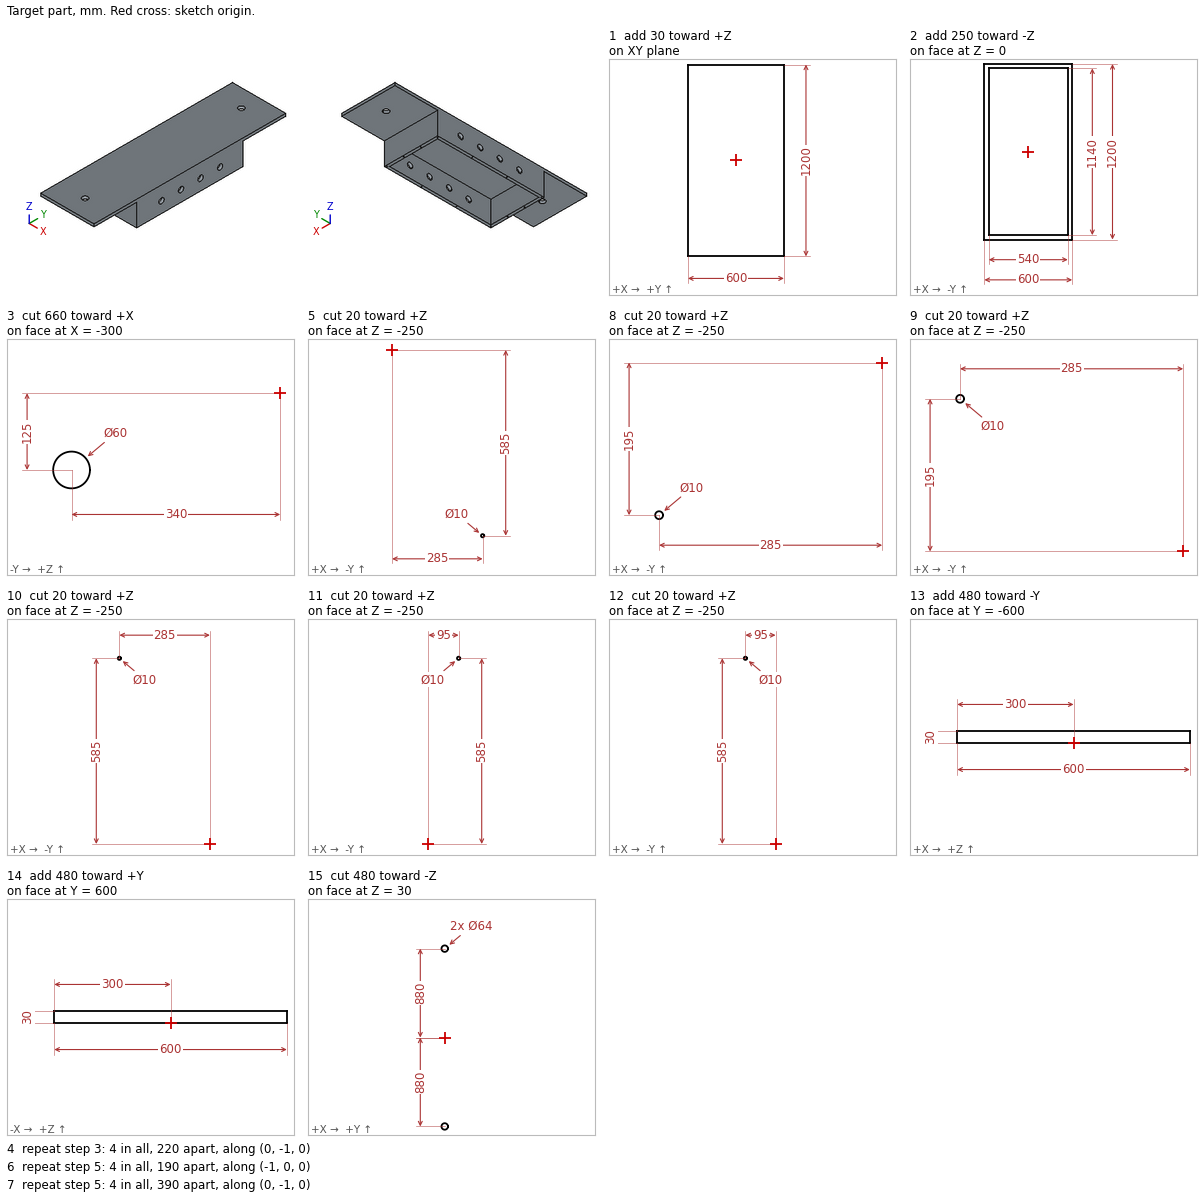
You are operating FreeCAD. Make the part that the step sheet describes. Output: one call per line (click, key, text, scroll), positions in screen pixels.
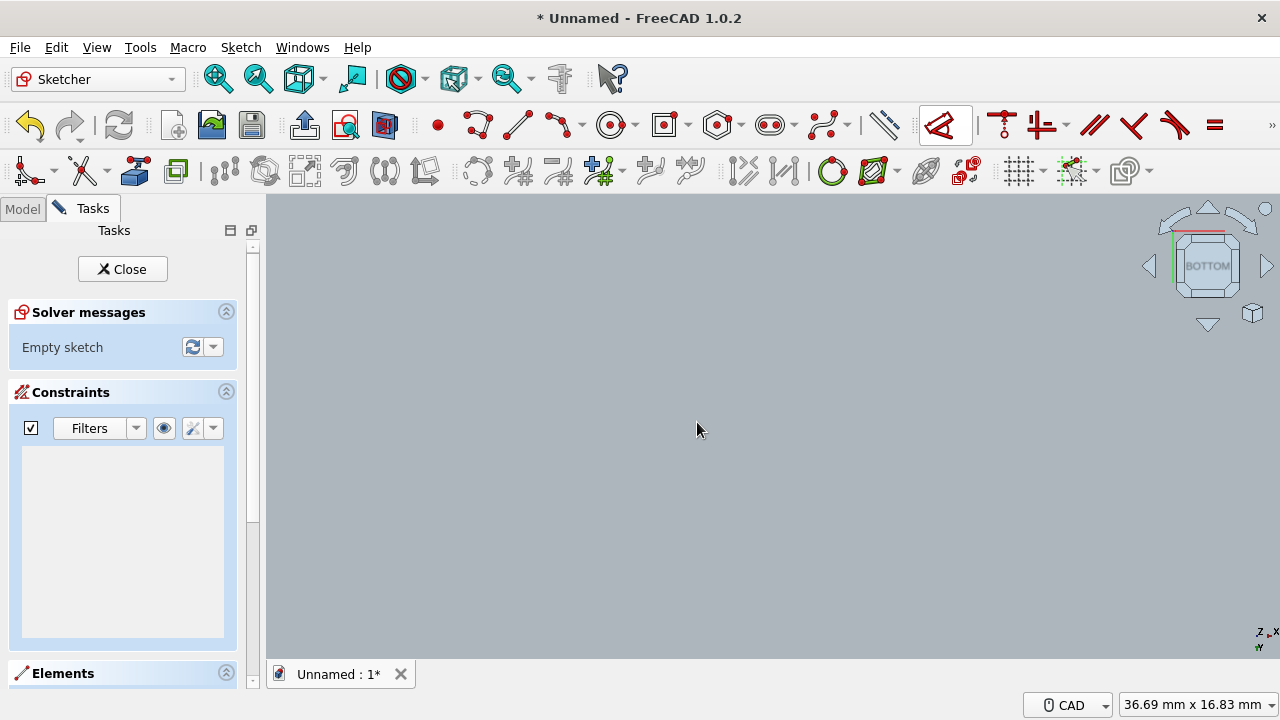
click(612, 126)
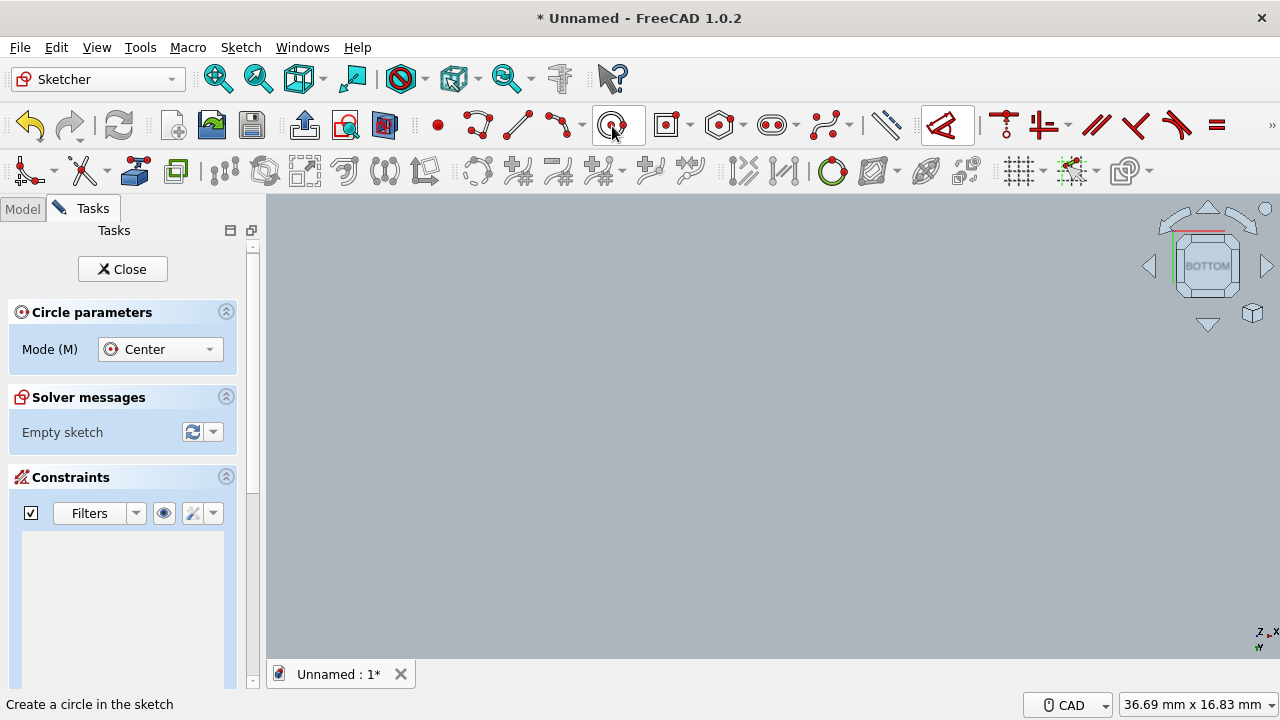
click(695, 418)
move(793, 320)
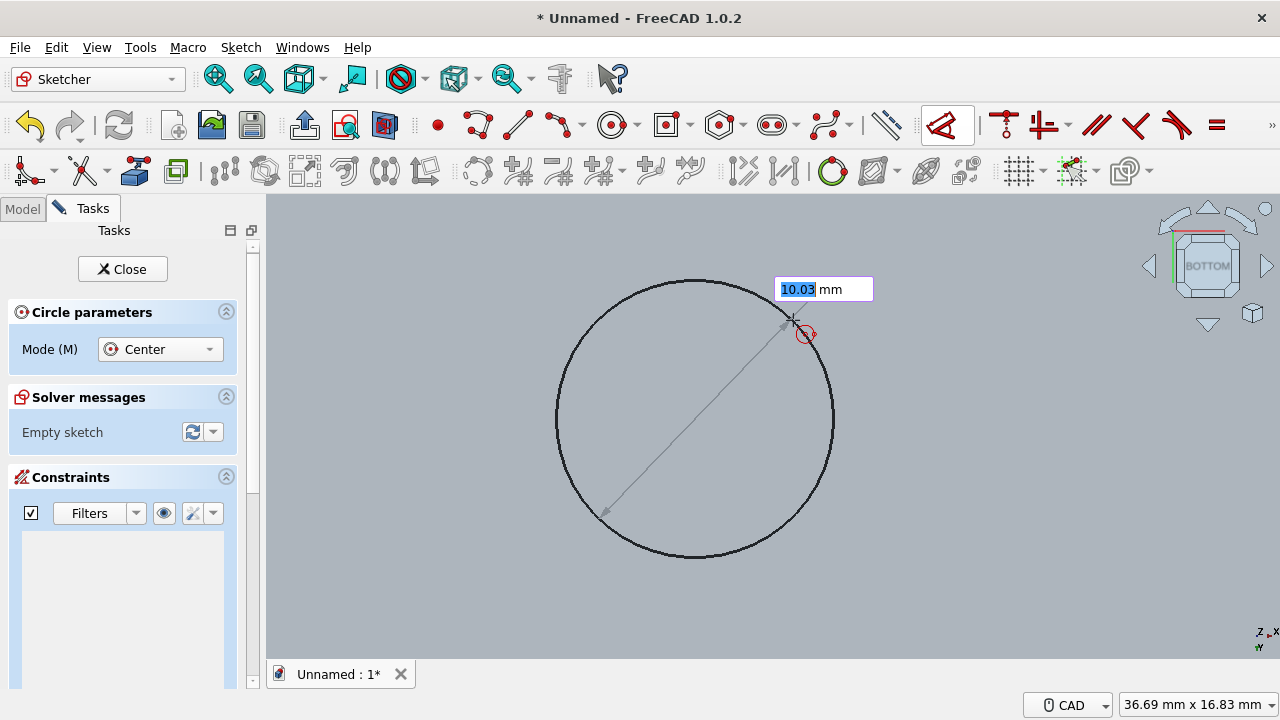
text(10)
key(Return)
key(Escape)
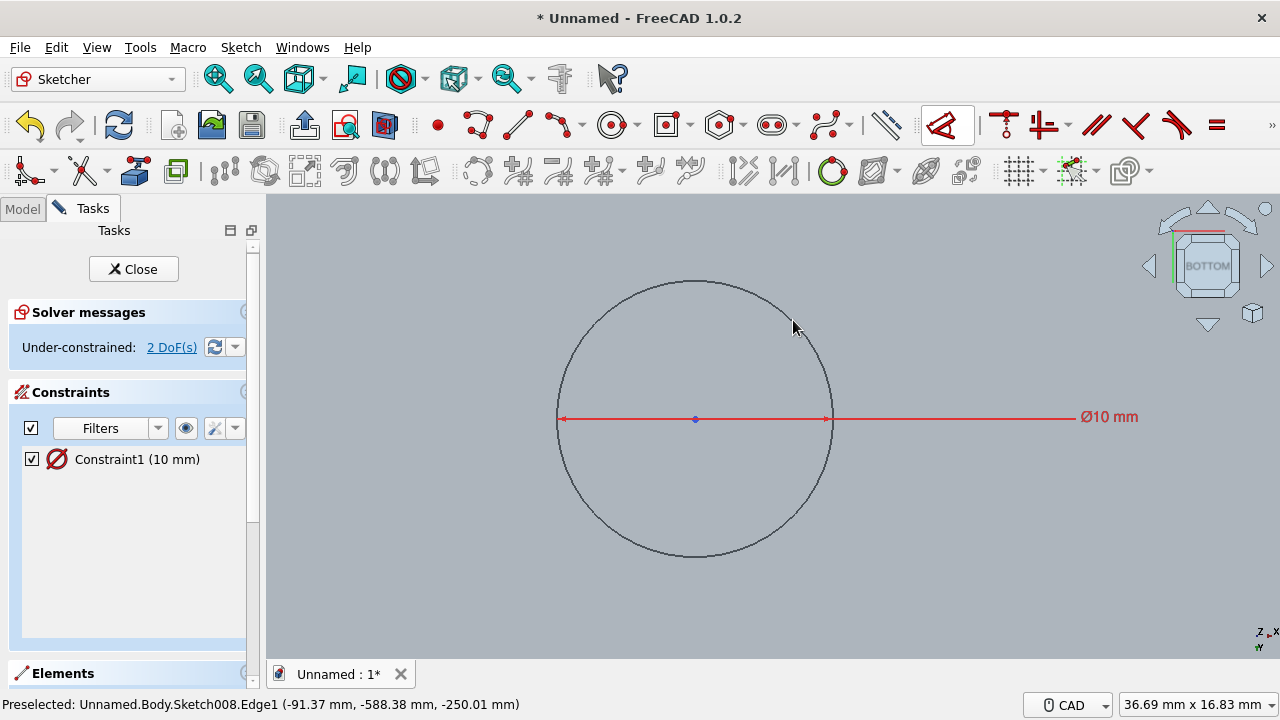
click(695, 419)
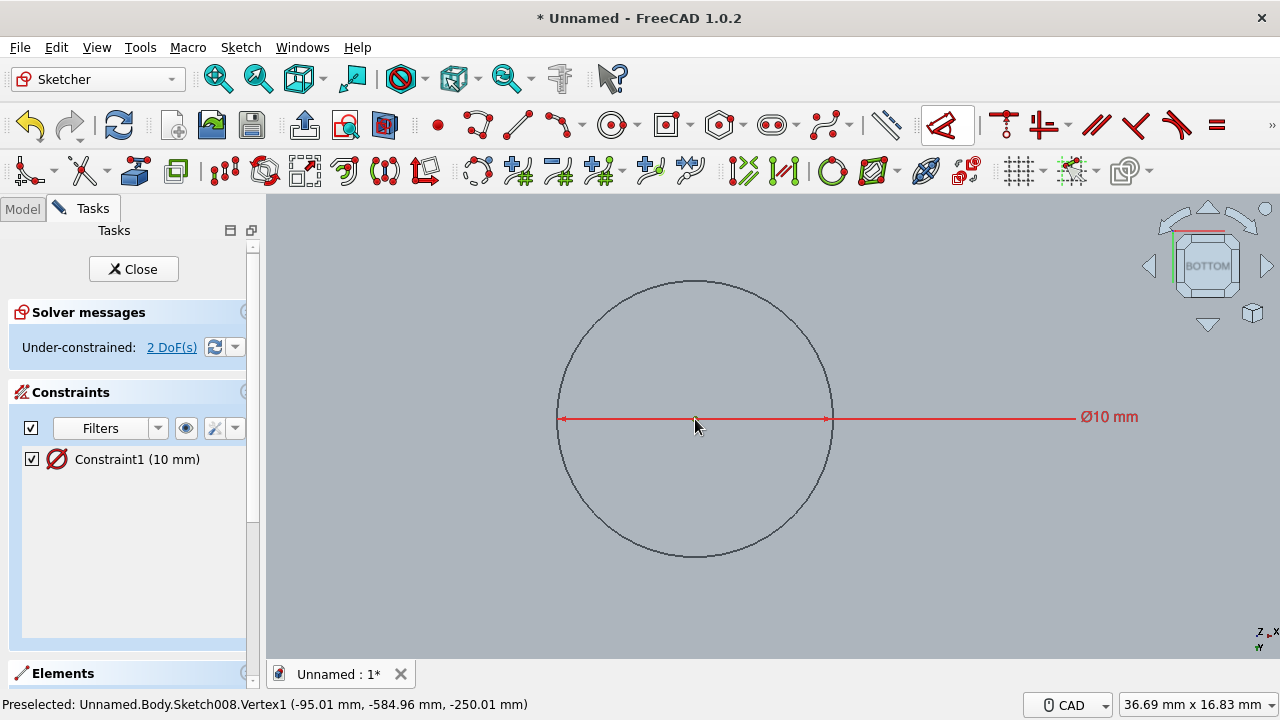
click(968, 126)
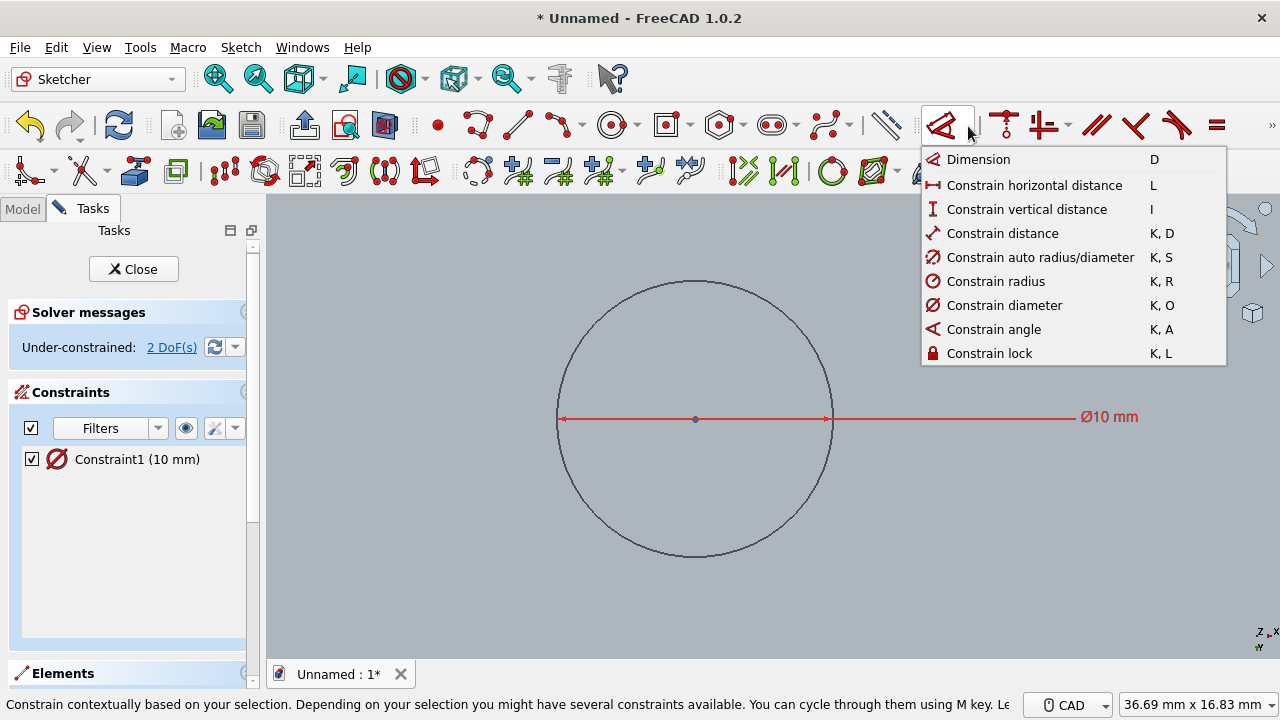
click(1074, 185)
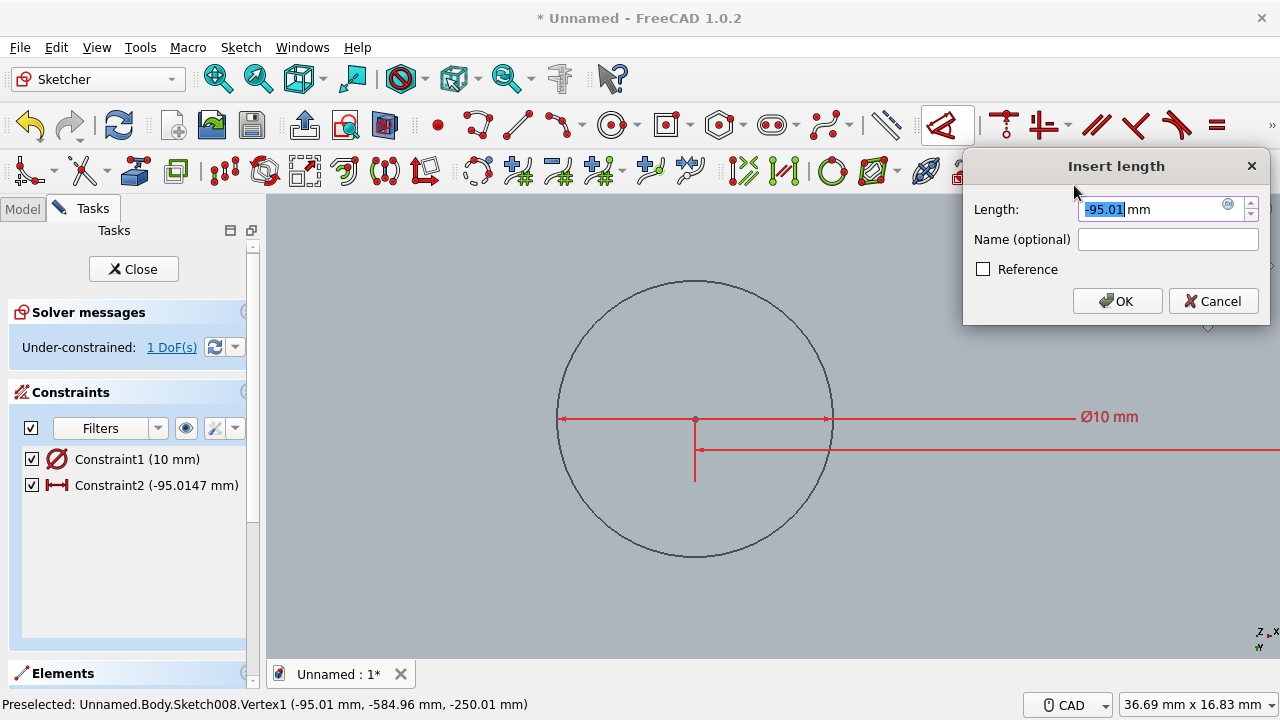
text(-95)
key(Return)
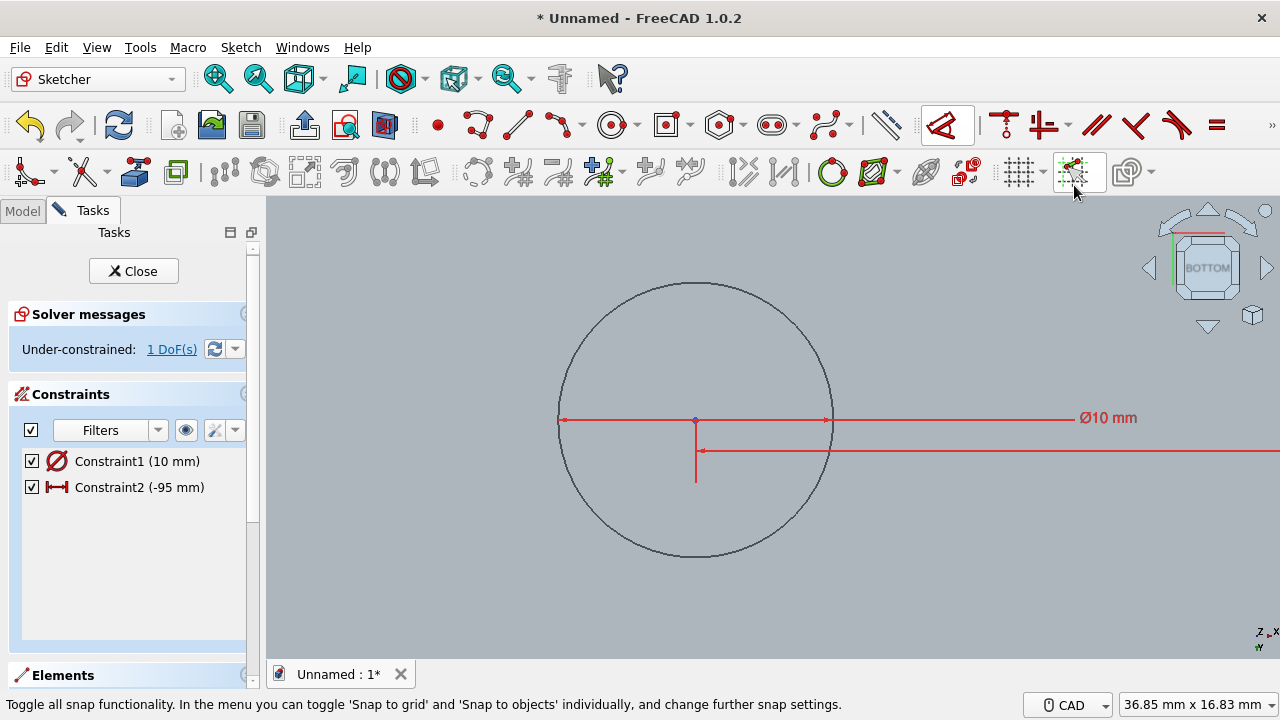
click(696, 420)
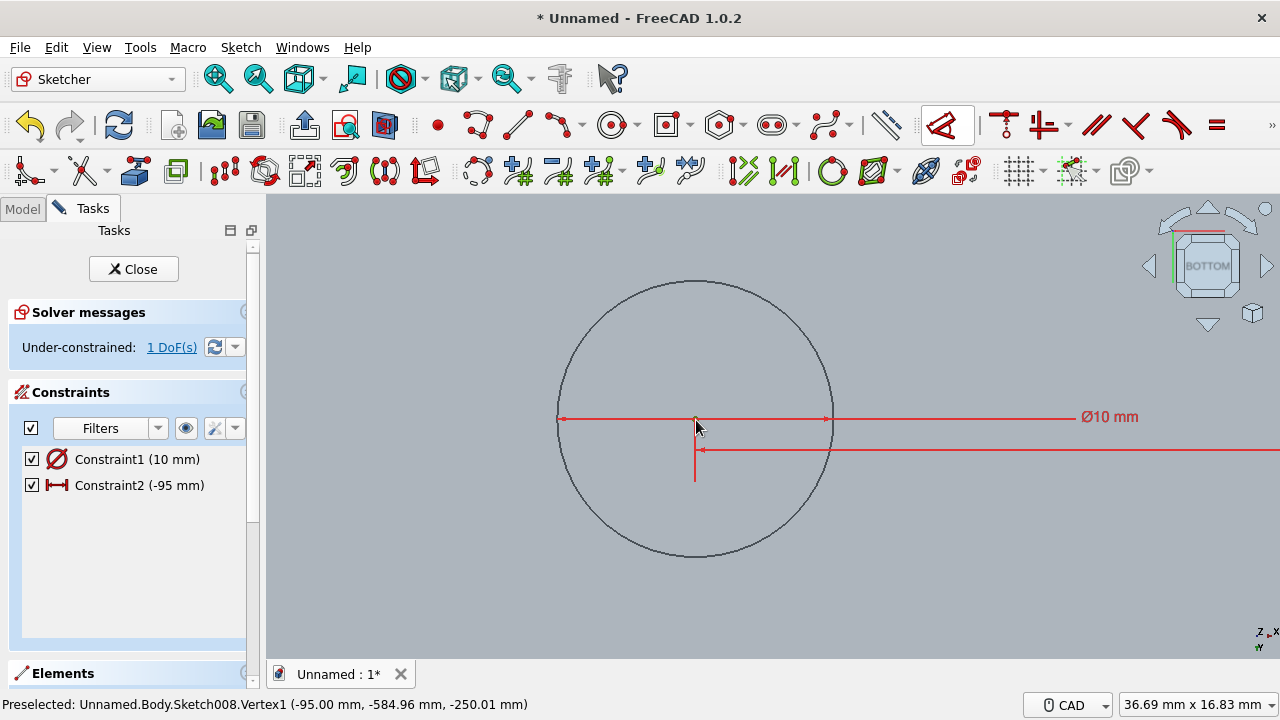
key(i)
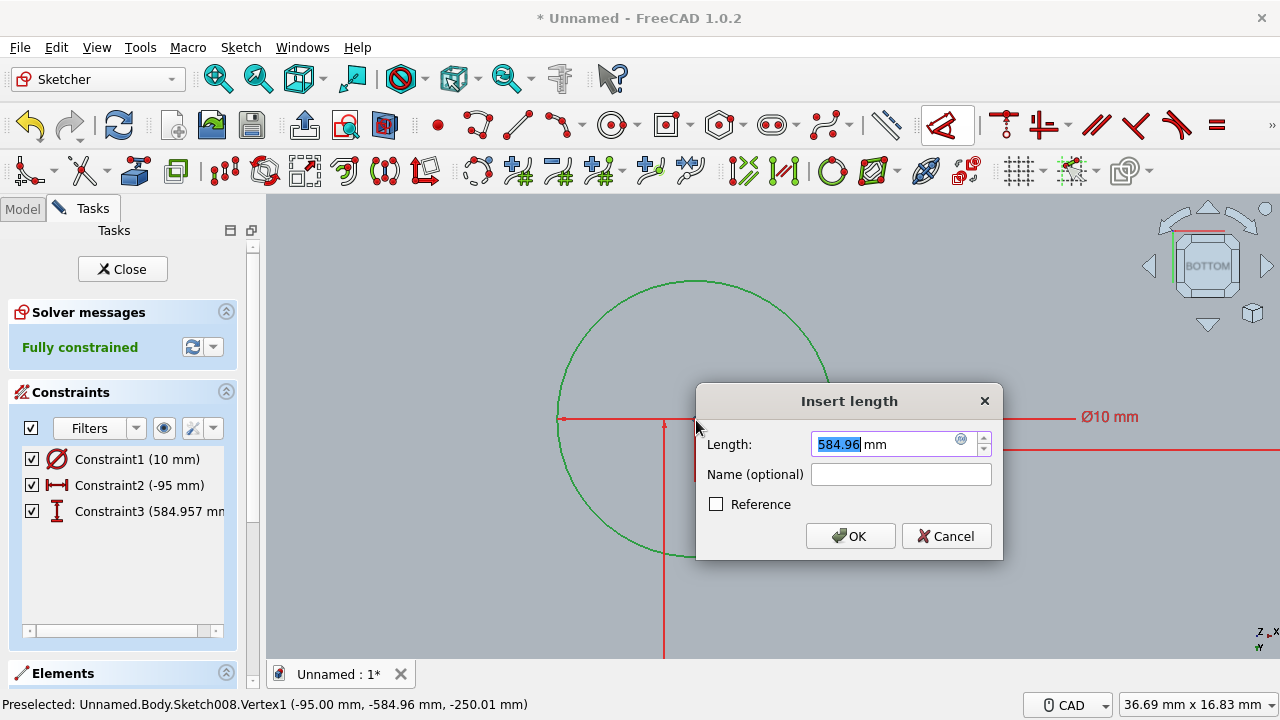
text(585)
key(Return)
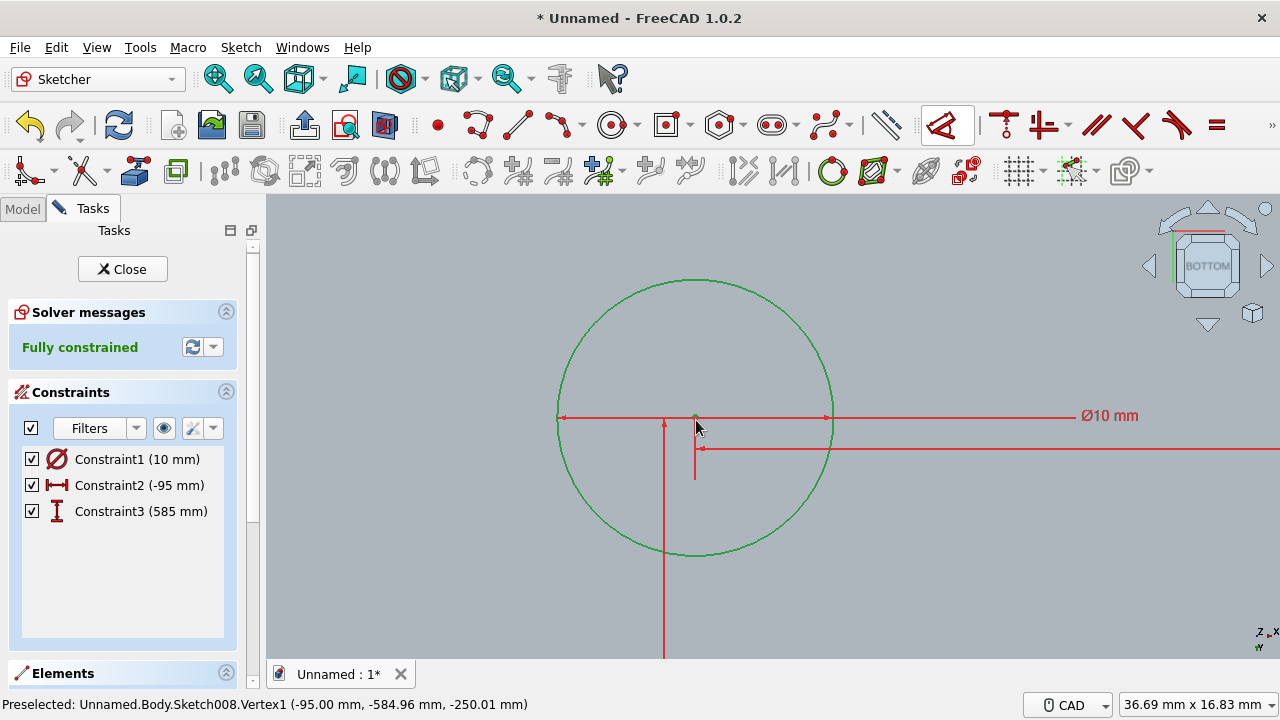
click(123, 269)